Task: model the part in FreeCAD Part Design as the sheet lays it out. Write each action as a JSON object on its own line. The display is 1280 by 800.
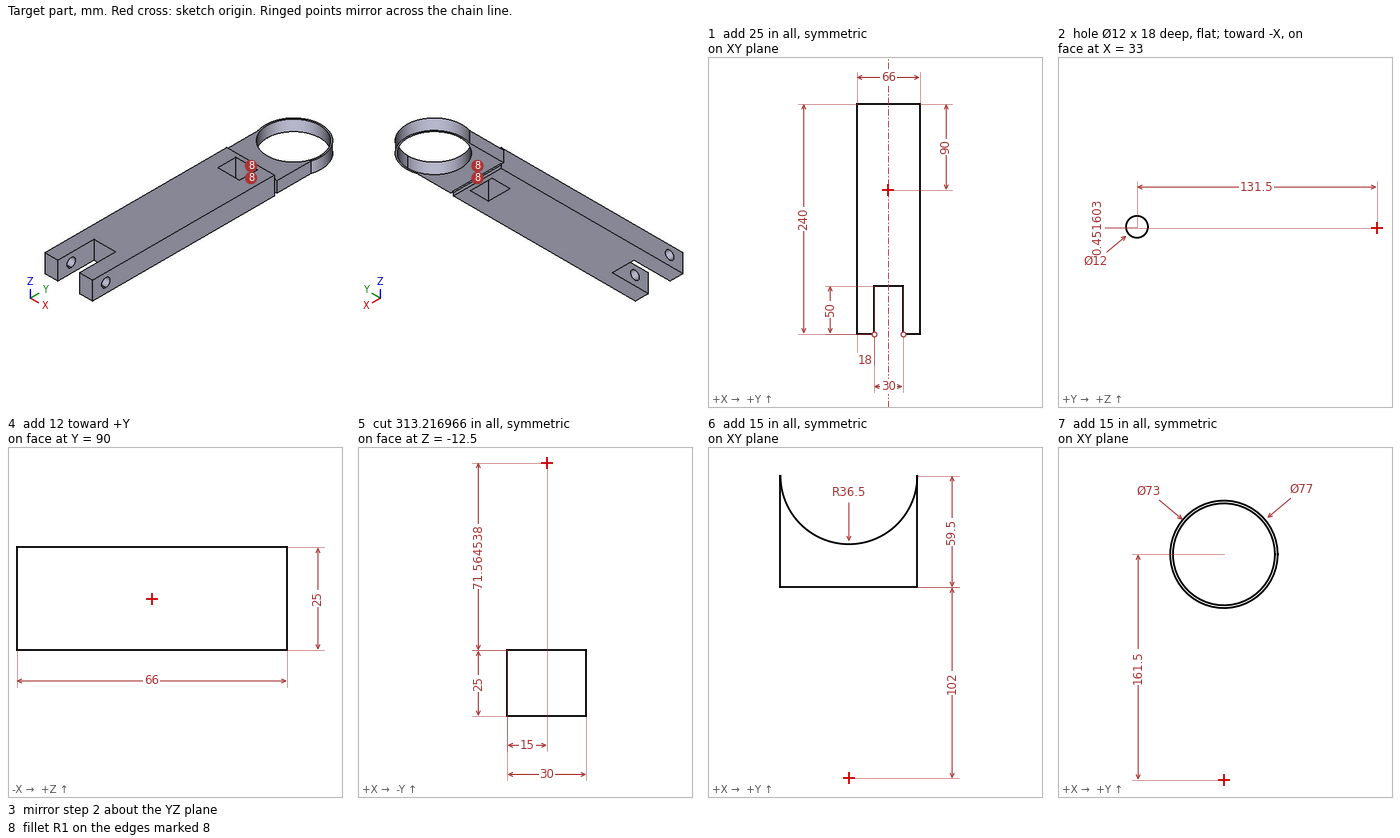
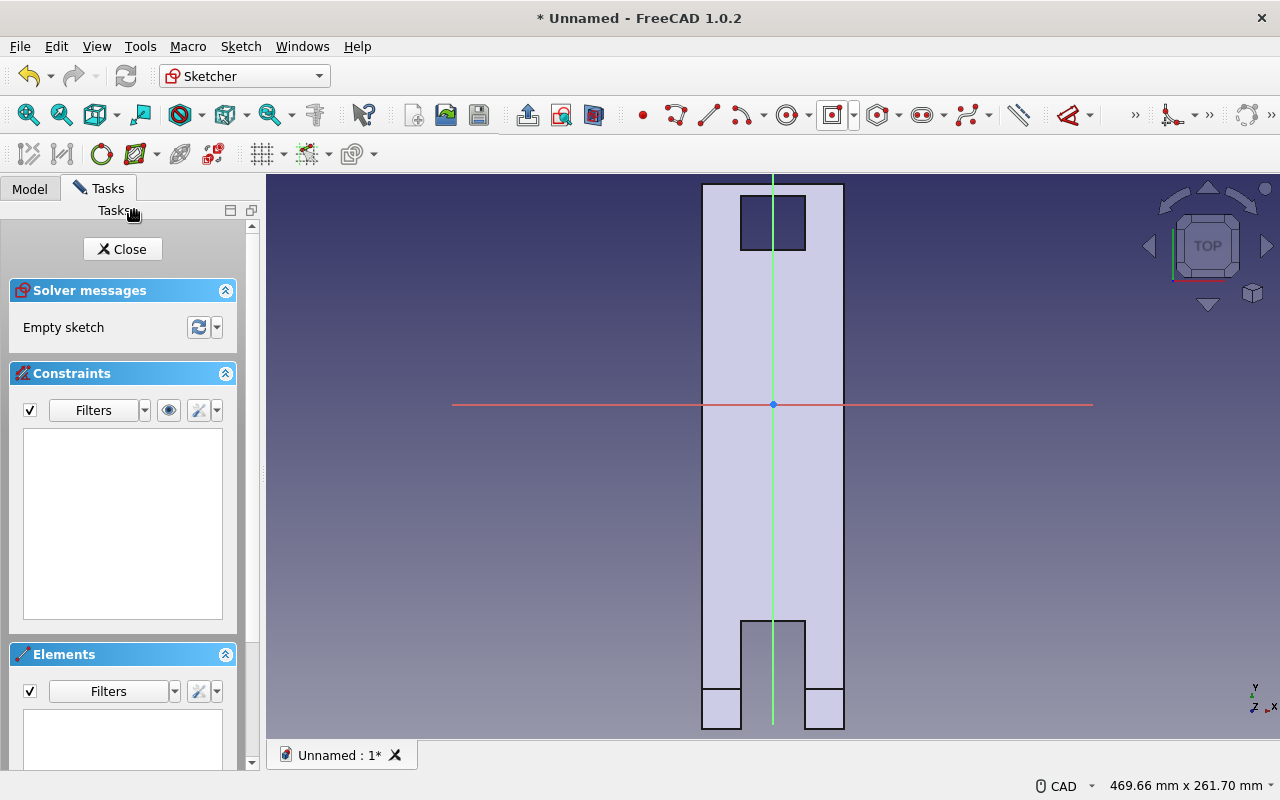
{"action": "scroll", "coordinate": [565, 711], "scroll_direction": "down", "scroll_amount": 2}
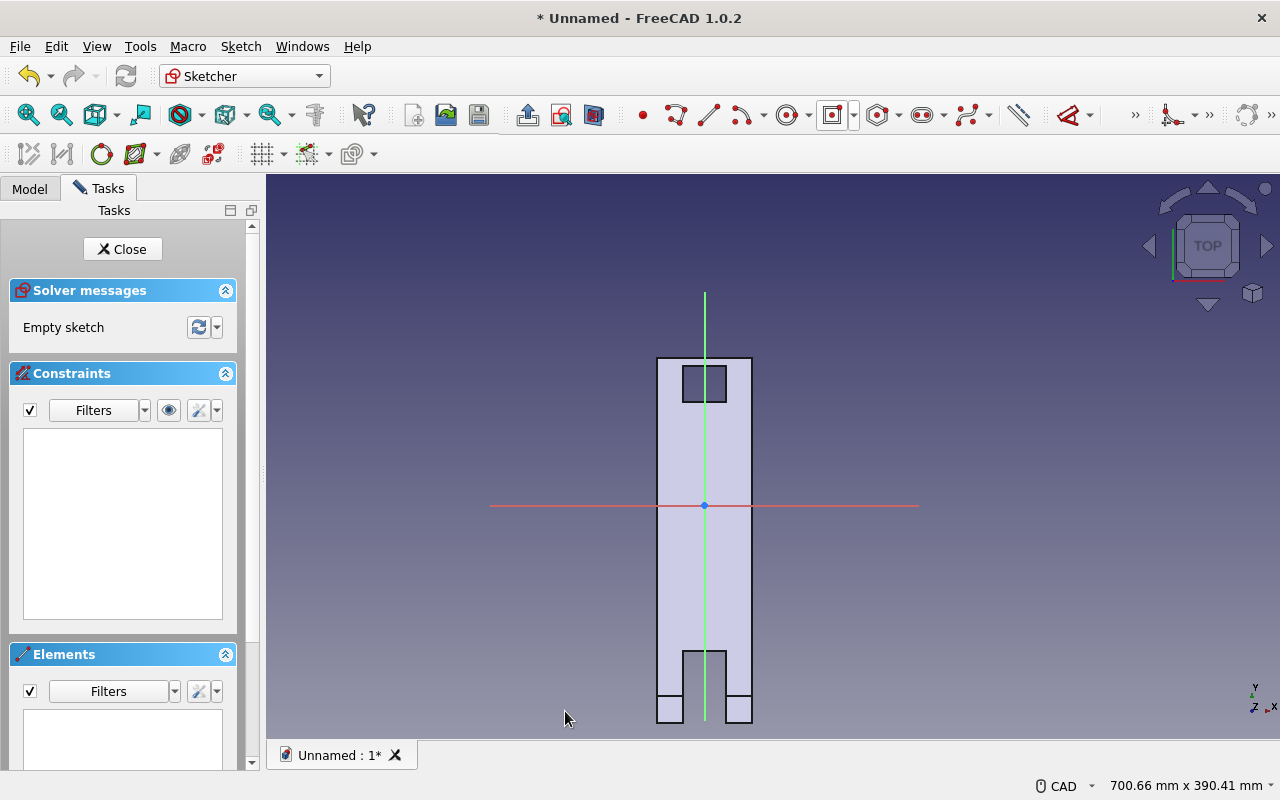
{"action": "scroll", "coordinate": [705, 252], "scroll_direction": "up", "scroll_amount": 2}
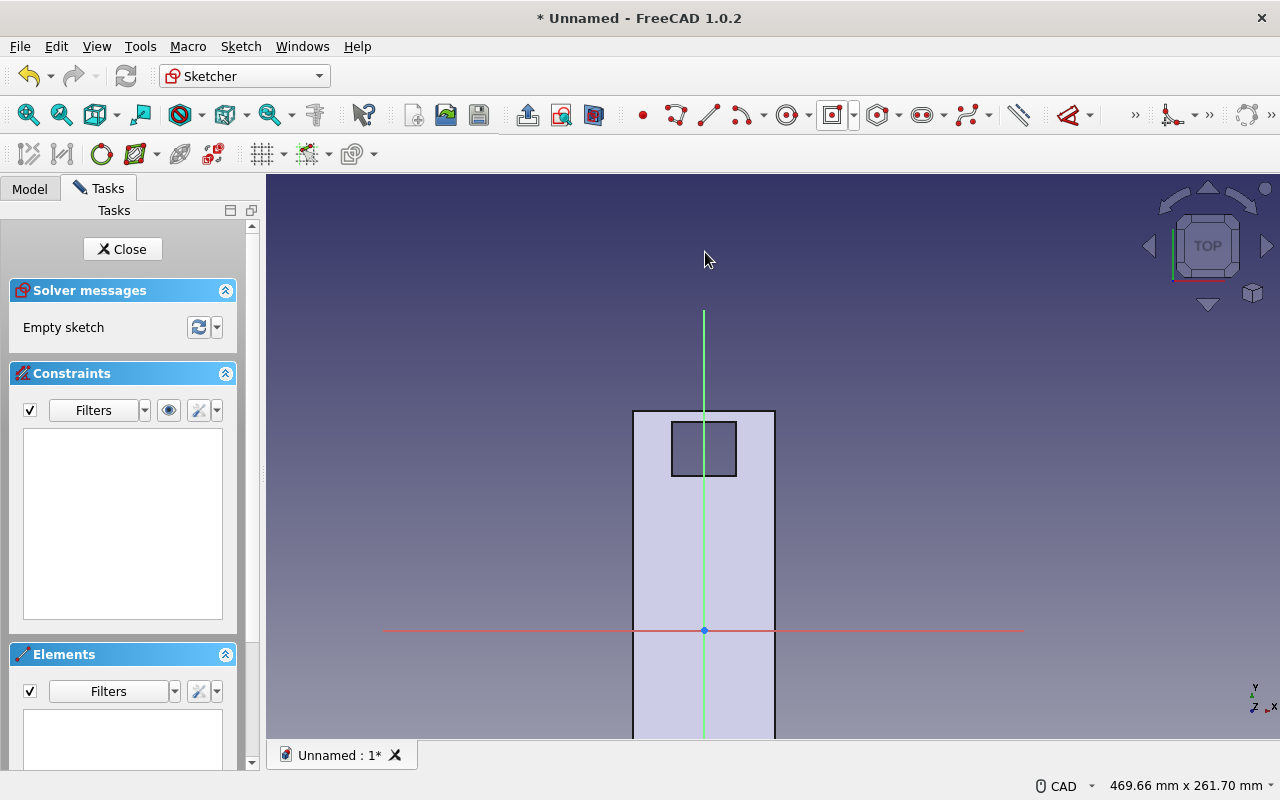
{"action": "key", "text": "g m"}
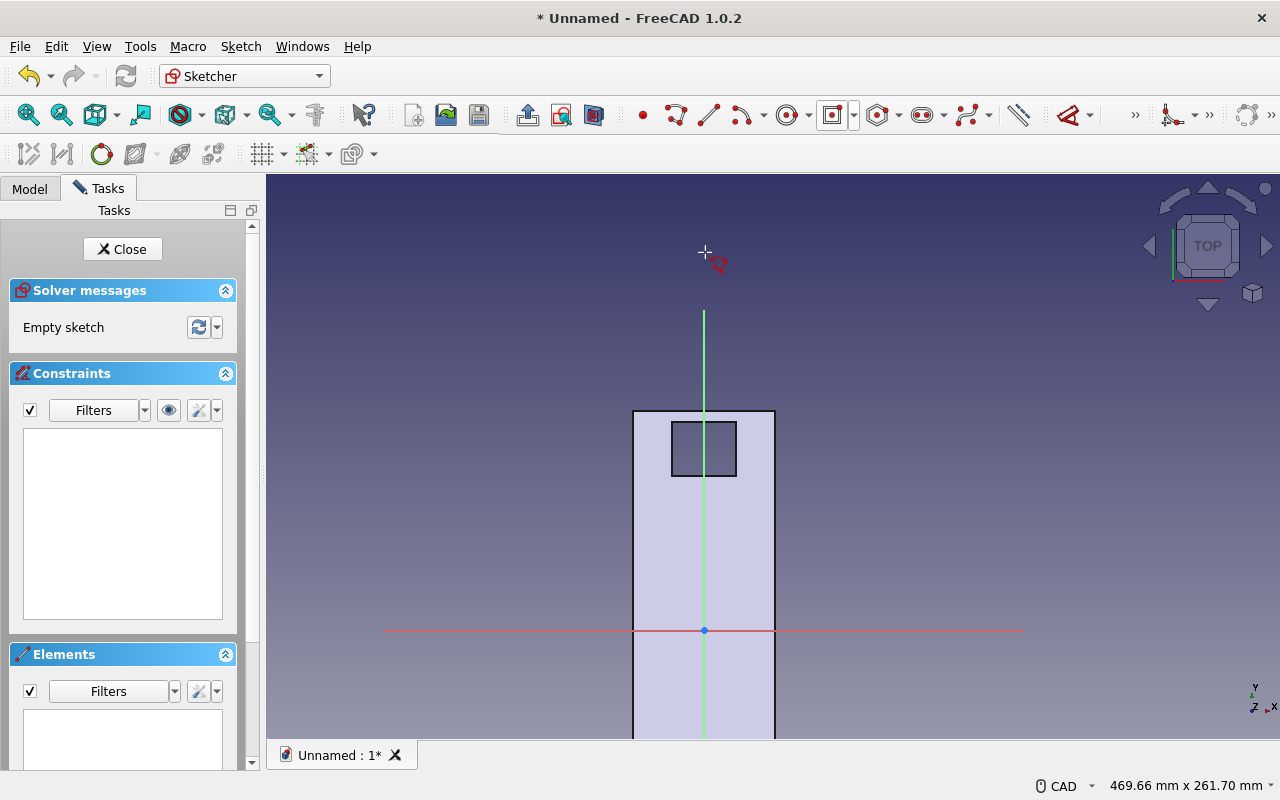
{"action": "left_click", "coordinate": [783, 282]}
{"action": "left_click", "coordinate": [783, 411]}
{"action": "left_click", "coordinate": [625, 411]}
{"action": "left_click", "coordinate": [625, 282]}
{"action": "right_click", "coordinate": [625, 282]}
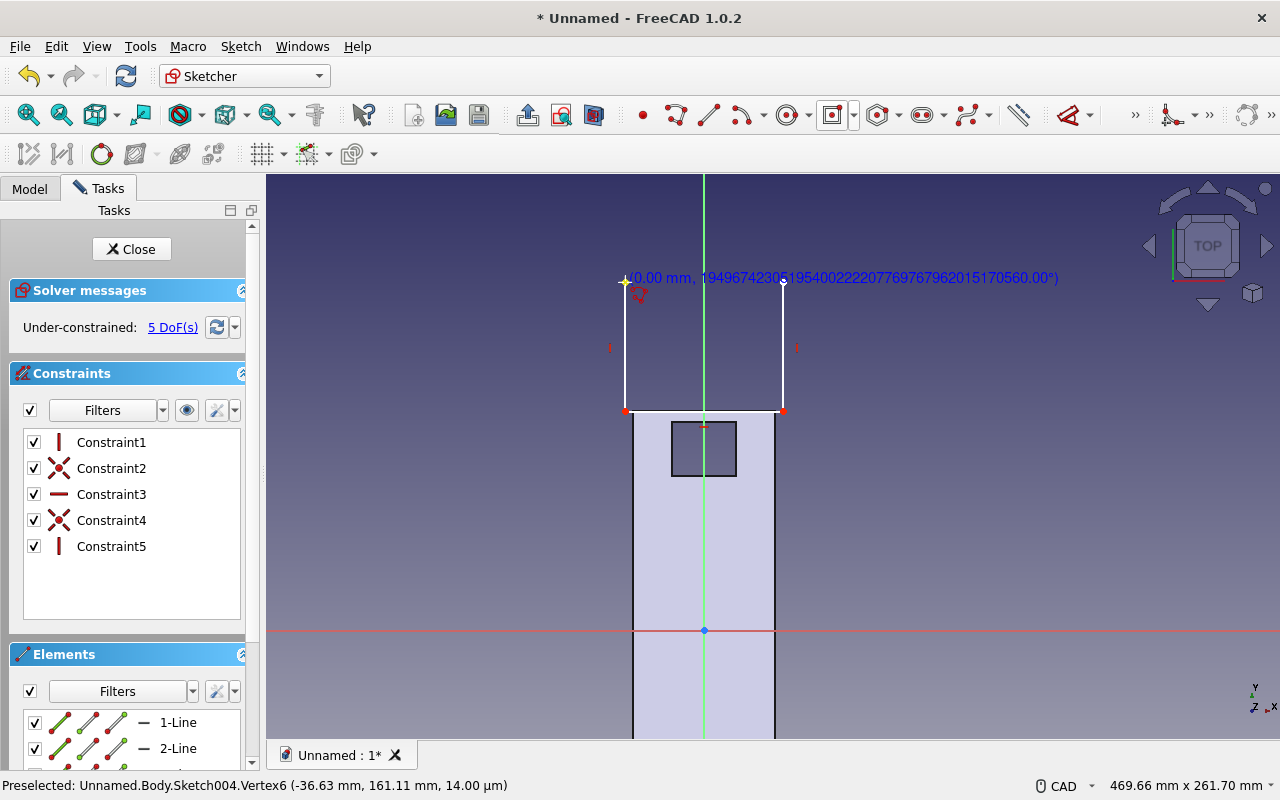
{"action": "left_click", "coordinate": [764, 116]}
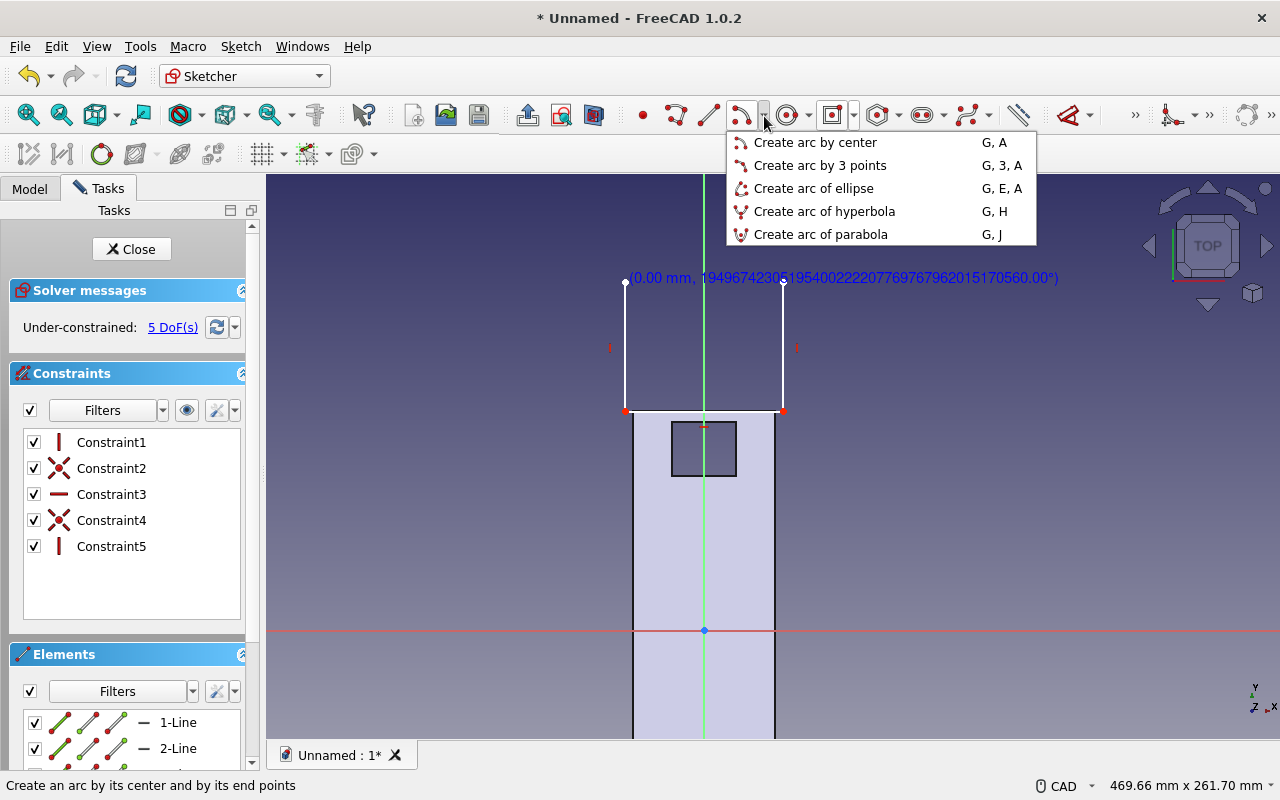
{"action": "left_click", "coordinate": [882, 166]}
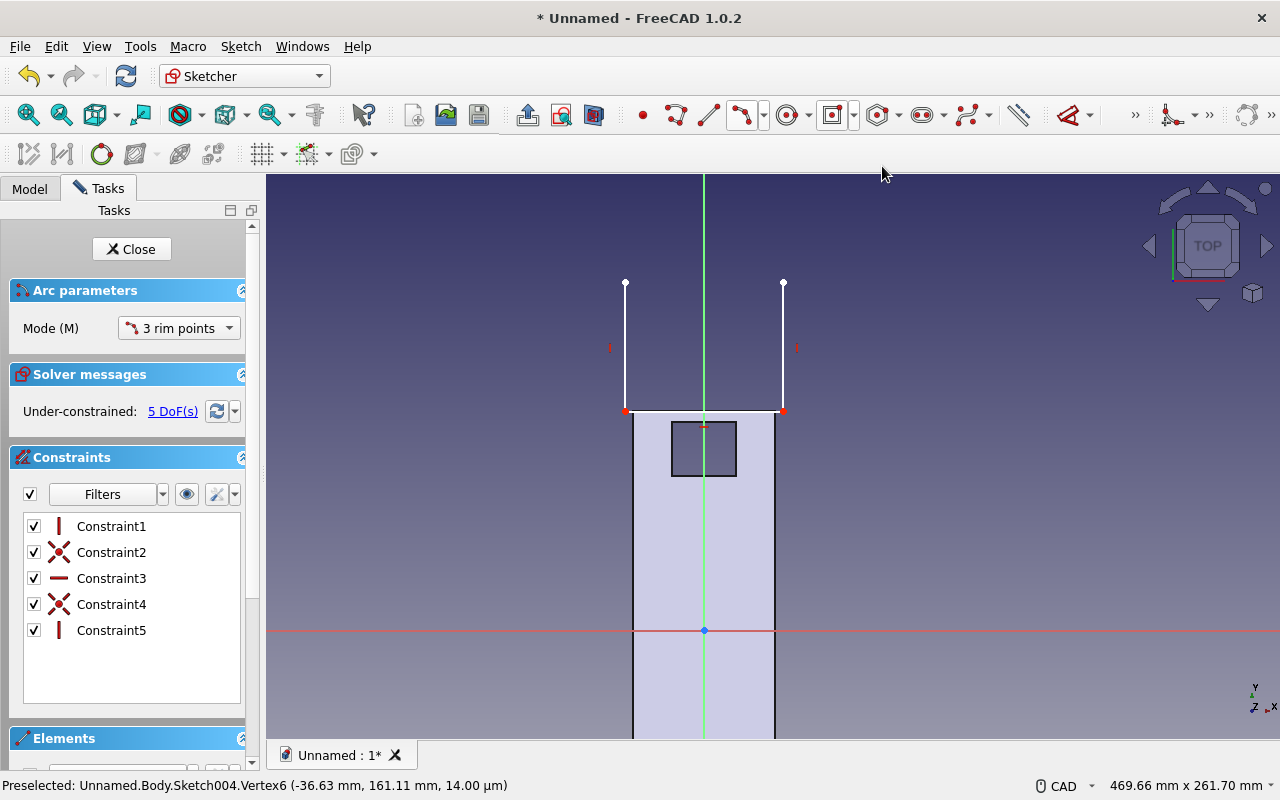
{"action": "left_click", "coordinate": [625, 283]}
{"action": "left_click", "coordinate": [783, 283]}
{"action": "left_click", "coordinate": [680, 357]}
{"action": "key", "text": "Escape"}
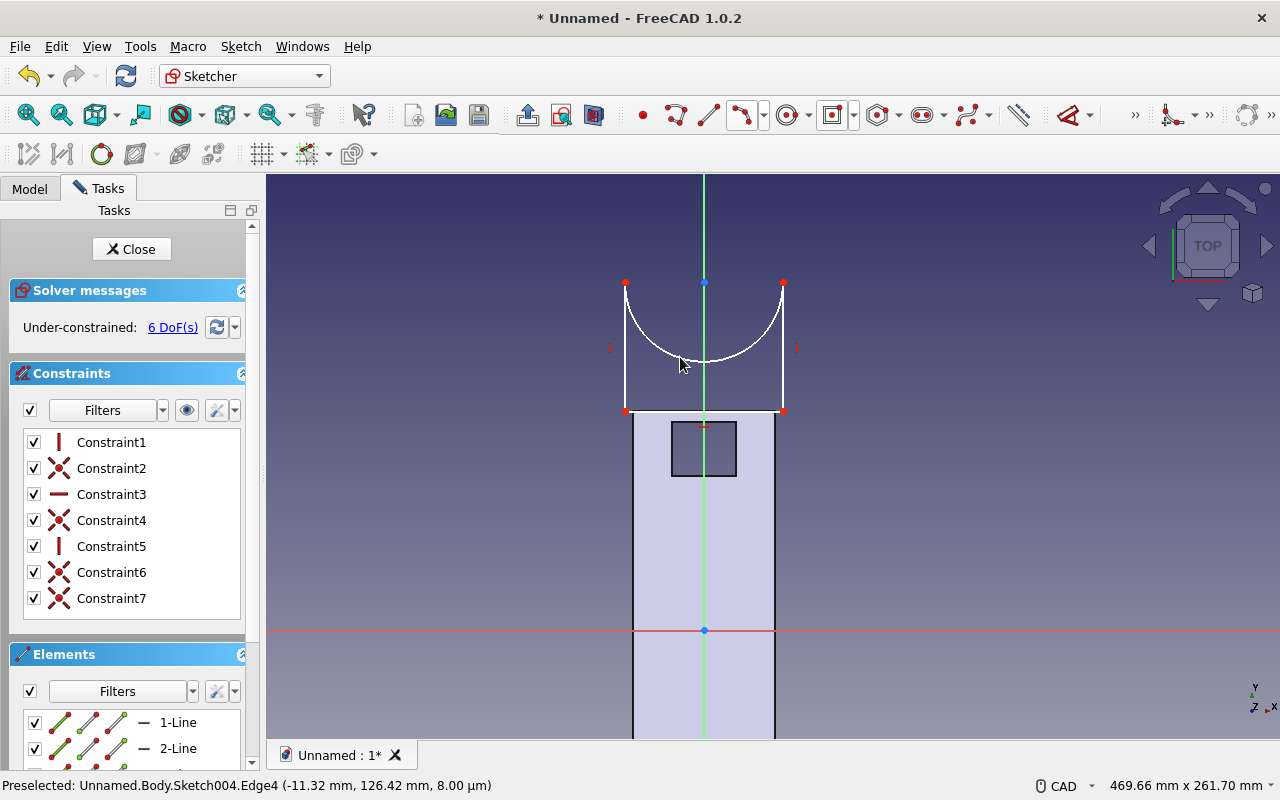
{"action": "scroll", "coordinate": [783, 322], "scroll_direction": "up", "scroll_amount": 3}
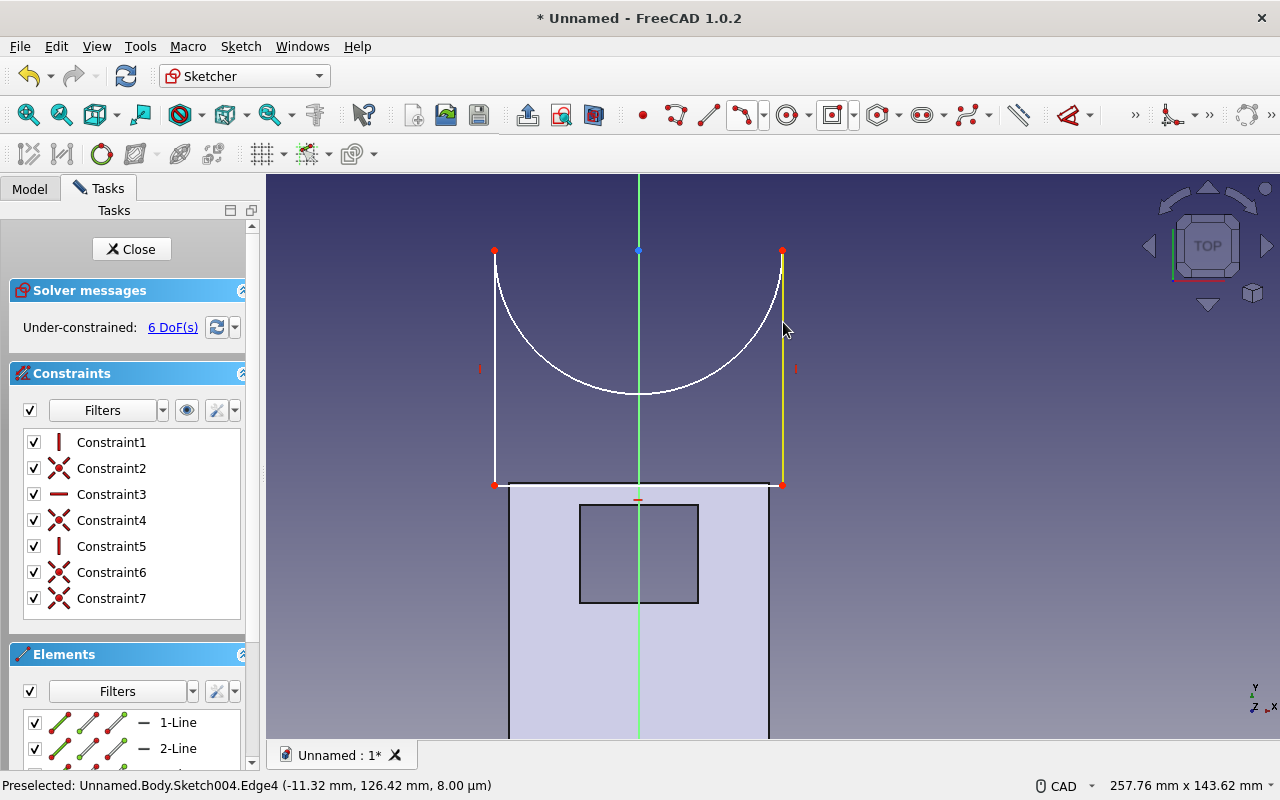
{"action": "left_click", "coordinate": [783, 321]}